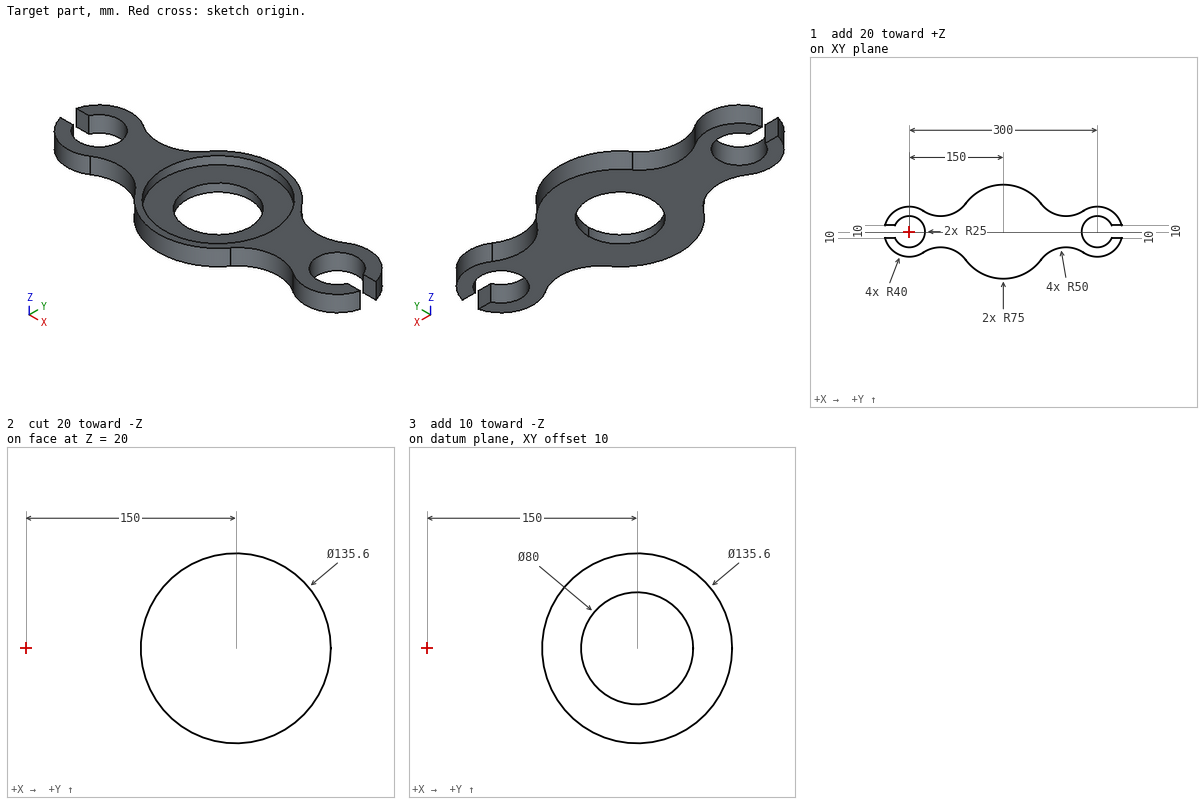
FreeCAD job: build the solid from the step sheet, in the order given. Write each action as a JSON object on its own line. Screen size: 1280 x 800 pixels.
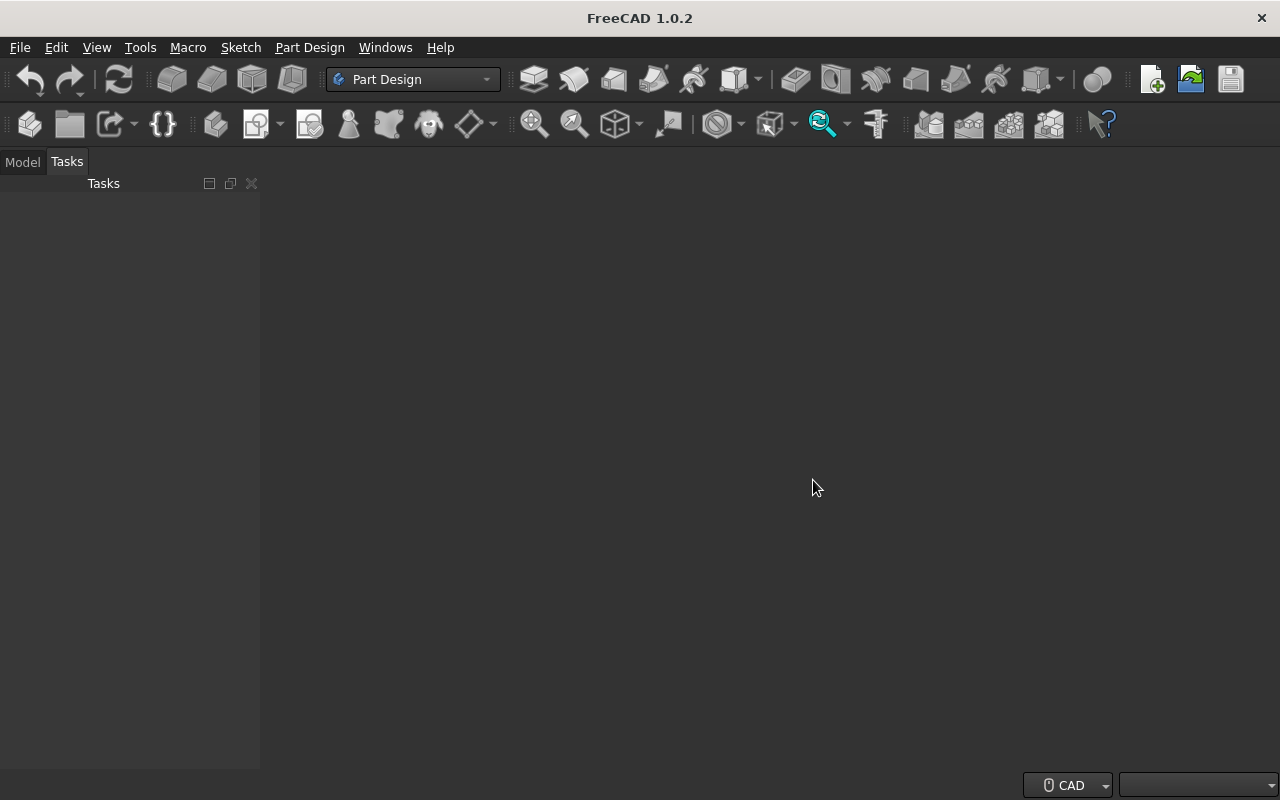
{"action": "left_click", "coordinate": [1152, 80]}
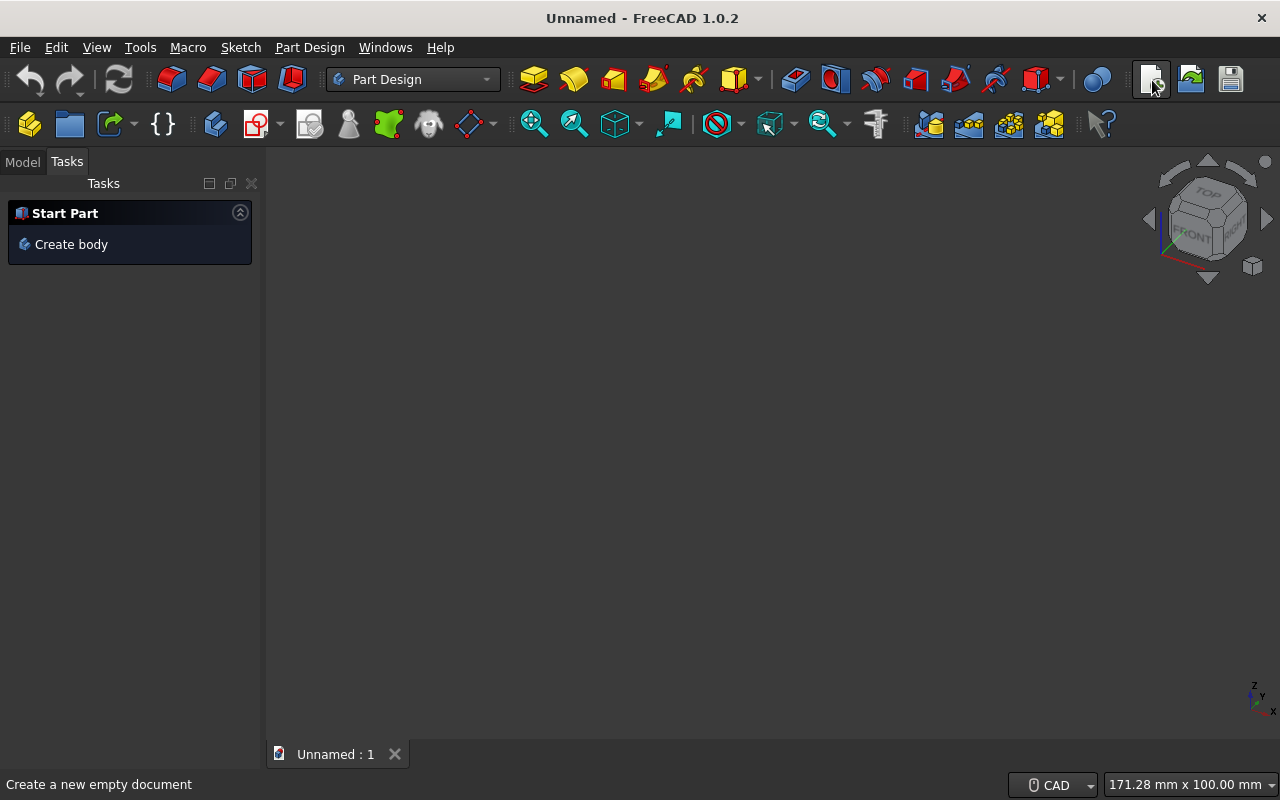
{"action": "left_click", "coordinate": [256, 124]}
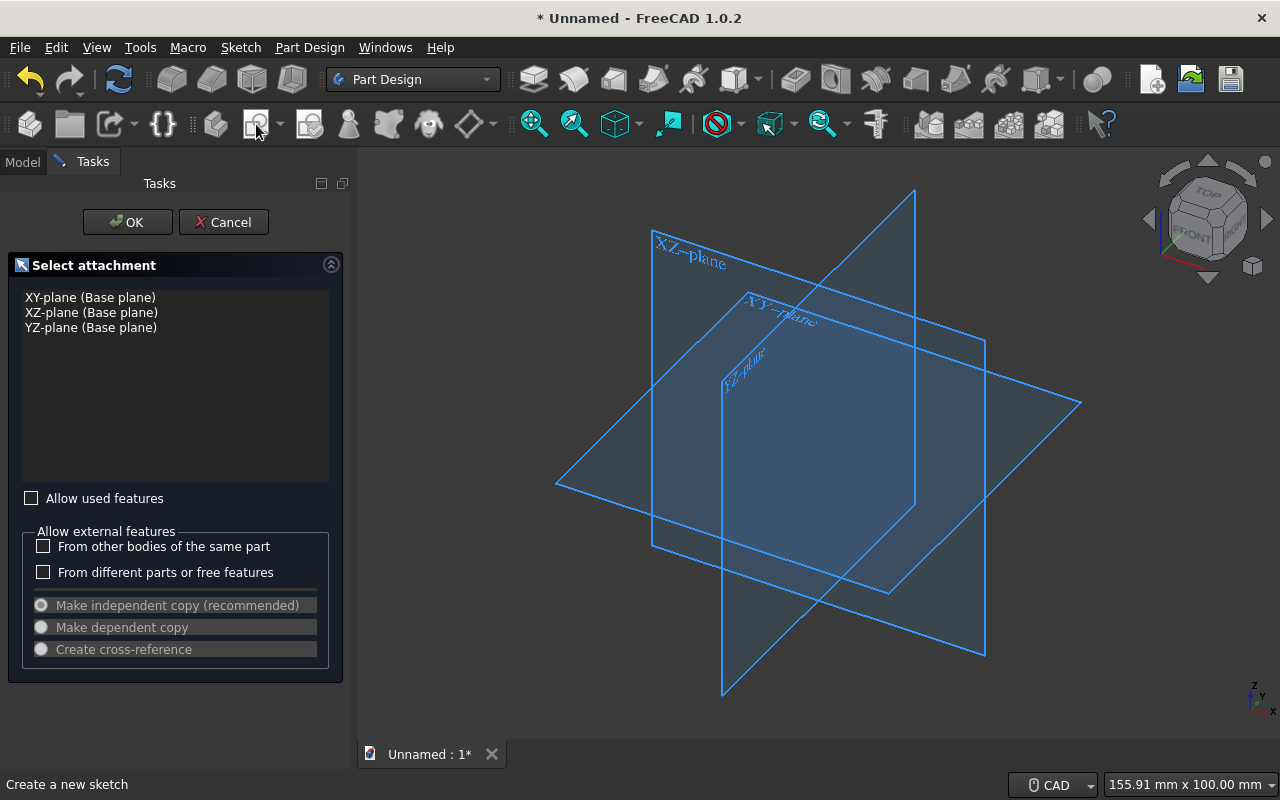
{"action": "left_click", "coordinate": [82, 298]}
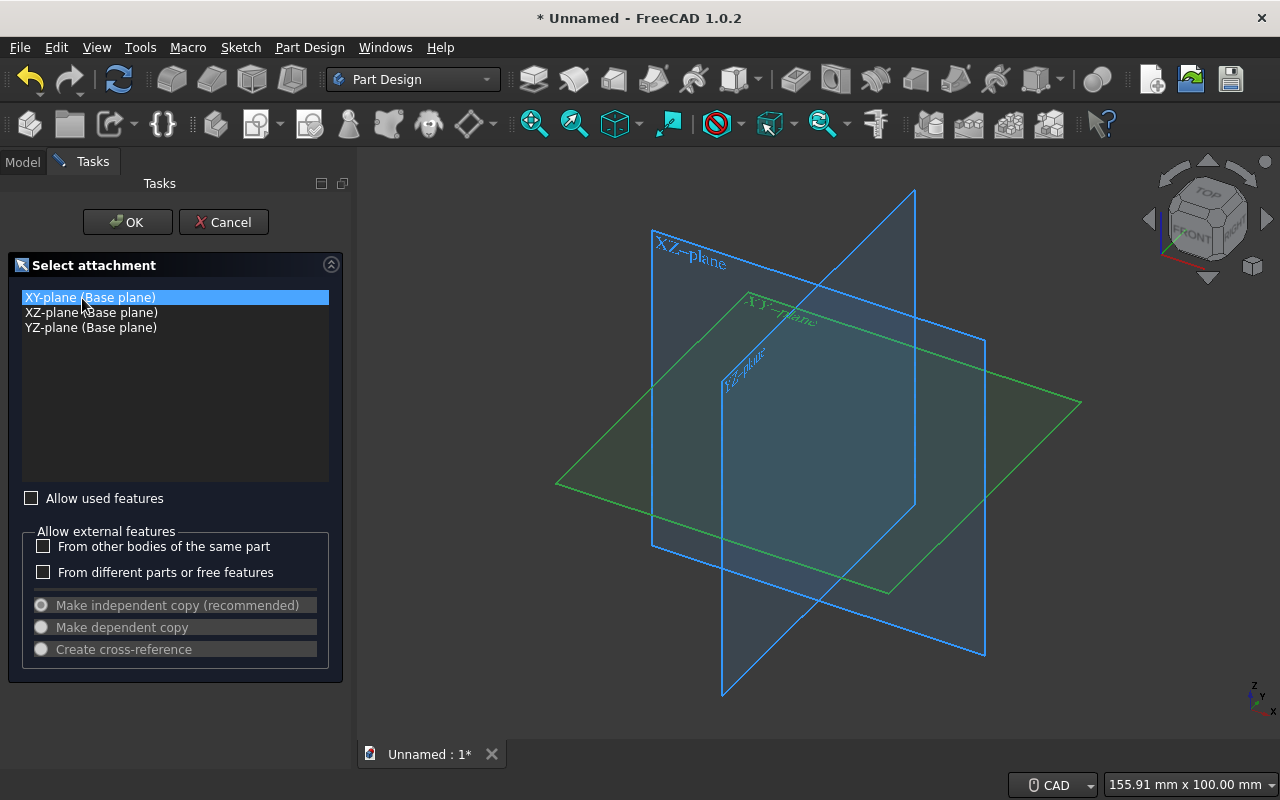
{"action": "left_click", "coordinate": [128, 222]}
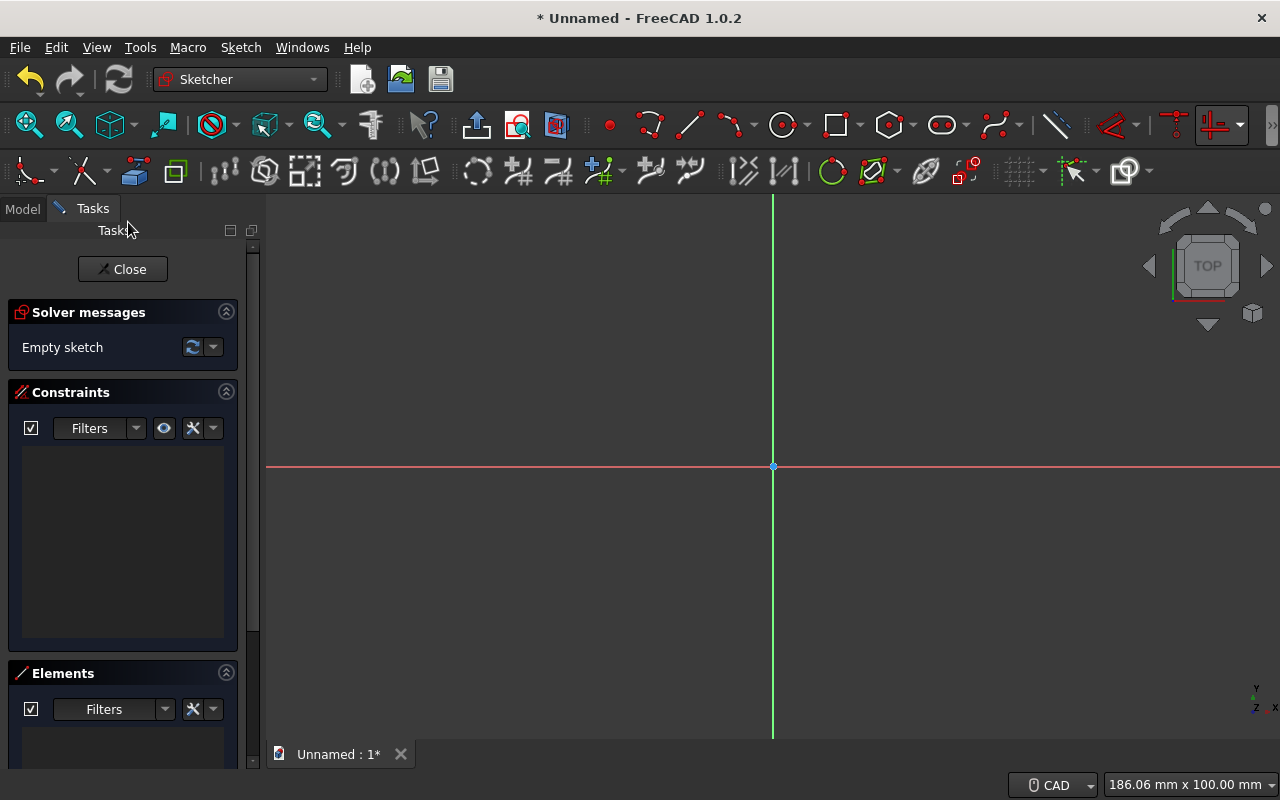
{"action": "scroll", "coordinate": [323, 466], "scroll_direction": "down", "scroll_amount": 6}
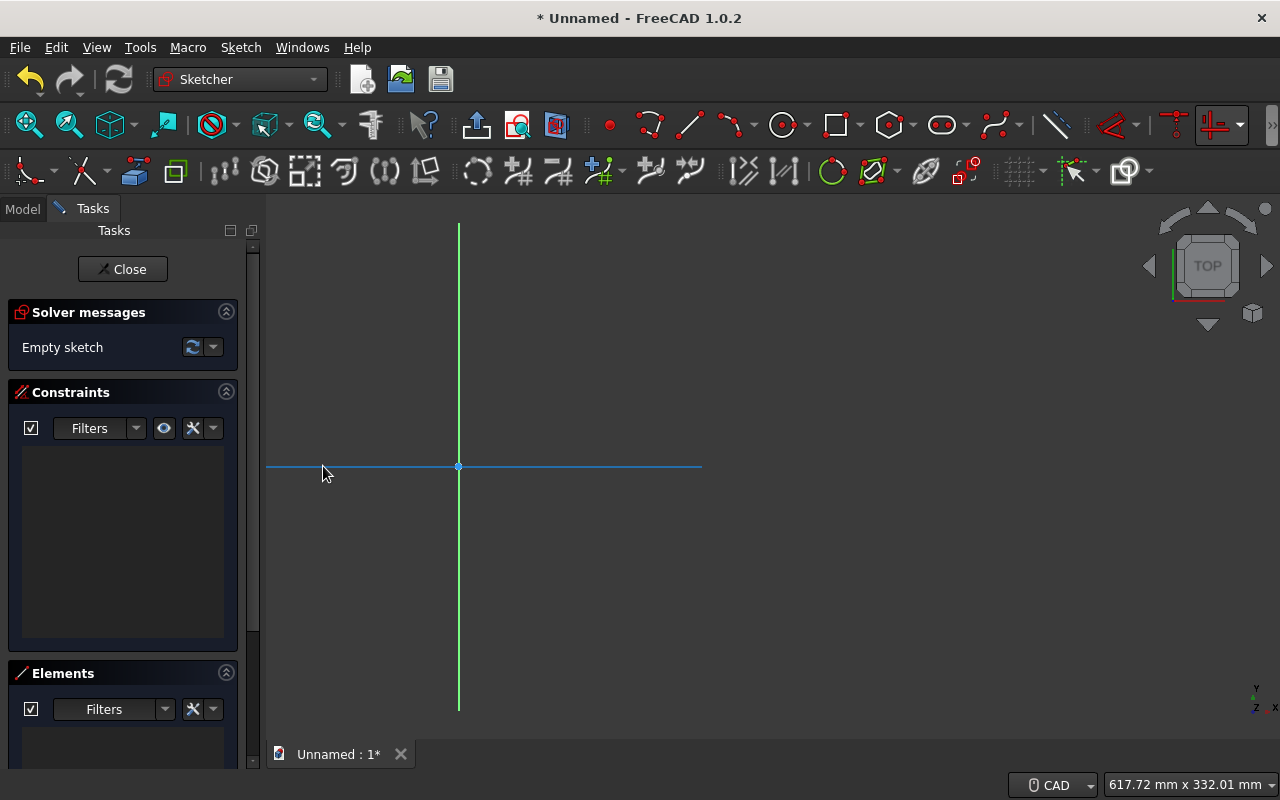
{"action": "left_click", "coordinate": [690, 126]}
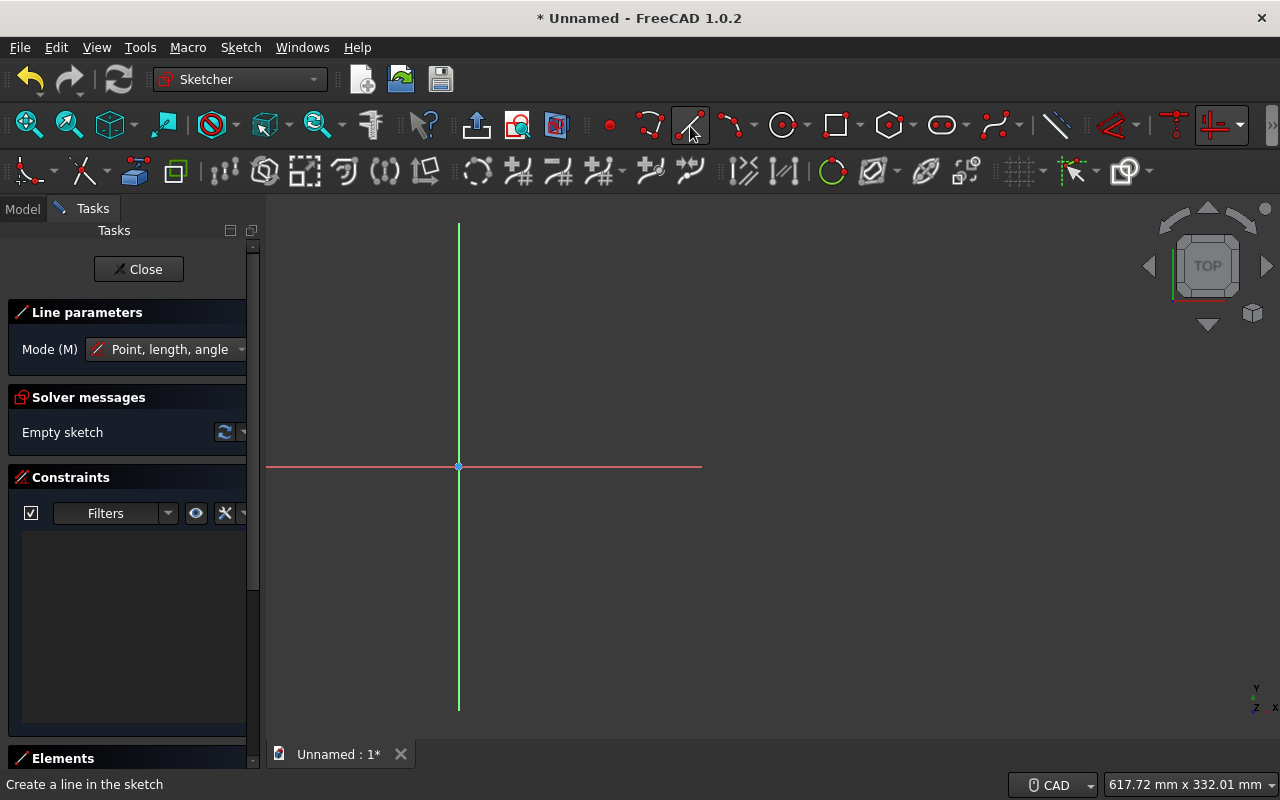
{"action": "left_click", "coordinate": [395, 450]}
{"action": "left_click", "coordinate": [421, 450]}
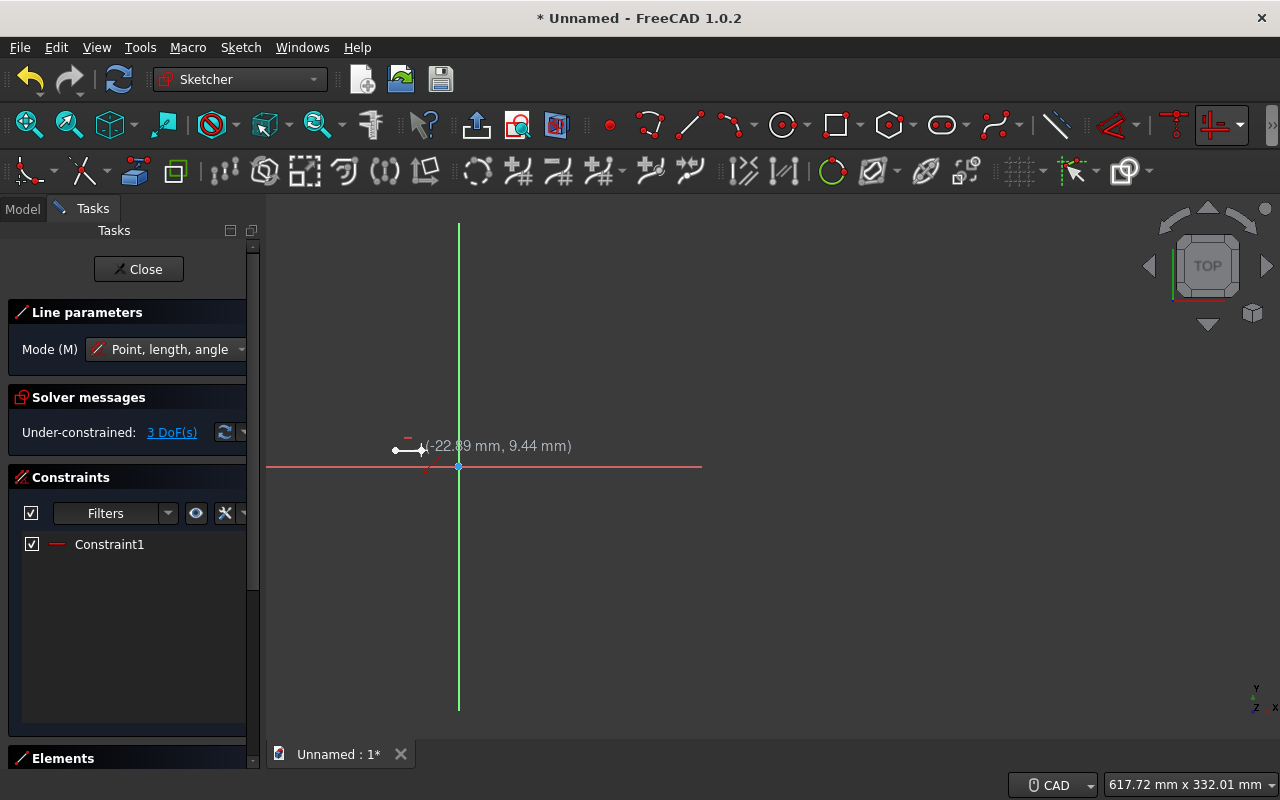
{"action": "left_click", "coordinate": [421, 483]}
{"action": "left_click", "coordinate": [395, 483]}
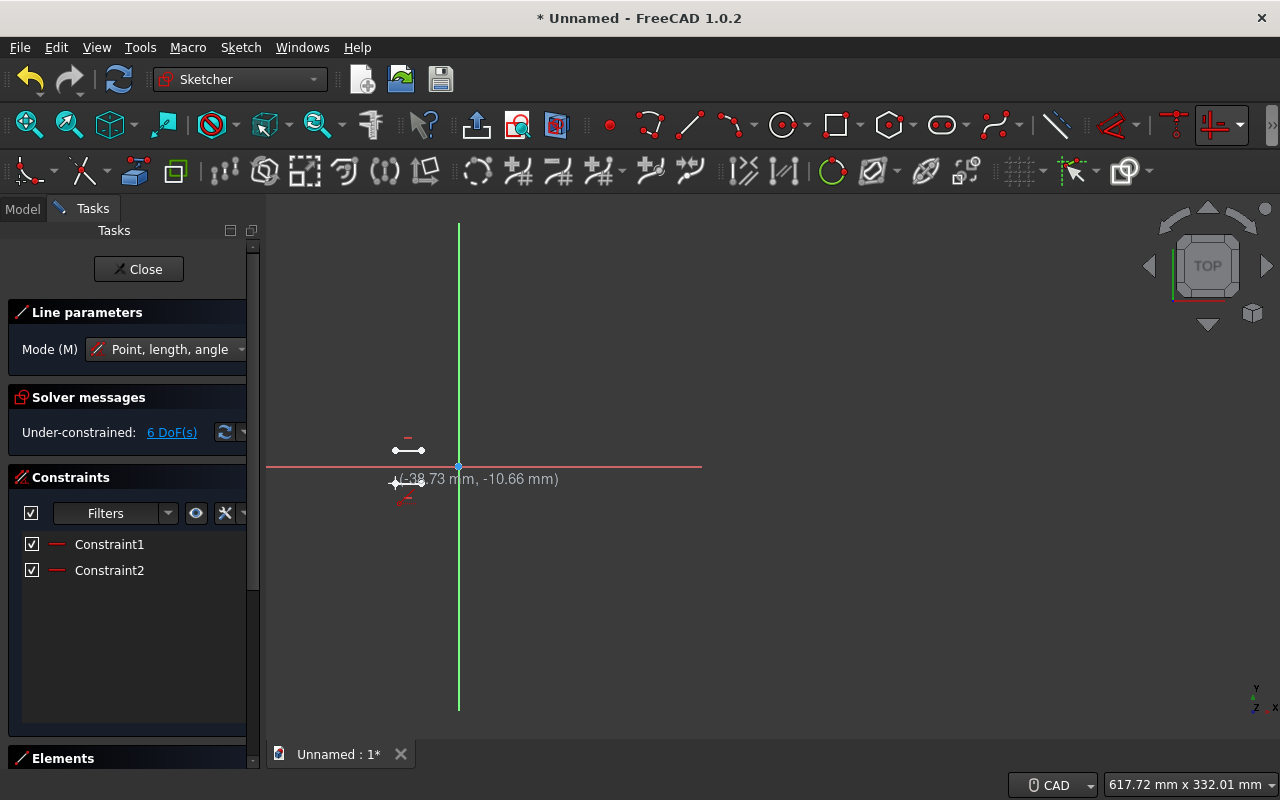
{"action": "left_click", "coordinate": [1015, 483]}
{"action": "left_click", "coordinate": [989, 483]}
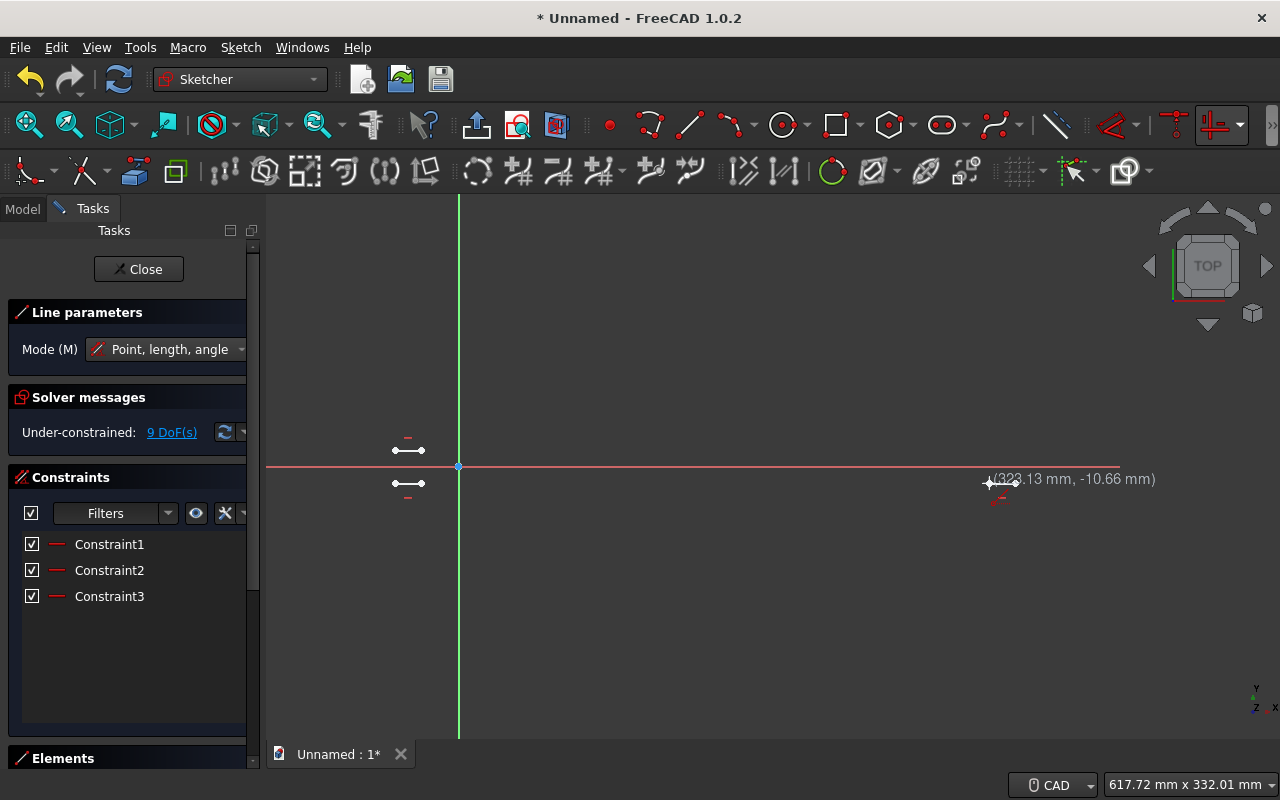
{"action": "left_click", "coordinate": [989, 450]}
{"action": "left_click", "coordinate": [1015, 450]}